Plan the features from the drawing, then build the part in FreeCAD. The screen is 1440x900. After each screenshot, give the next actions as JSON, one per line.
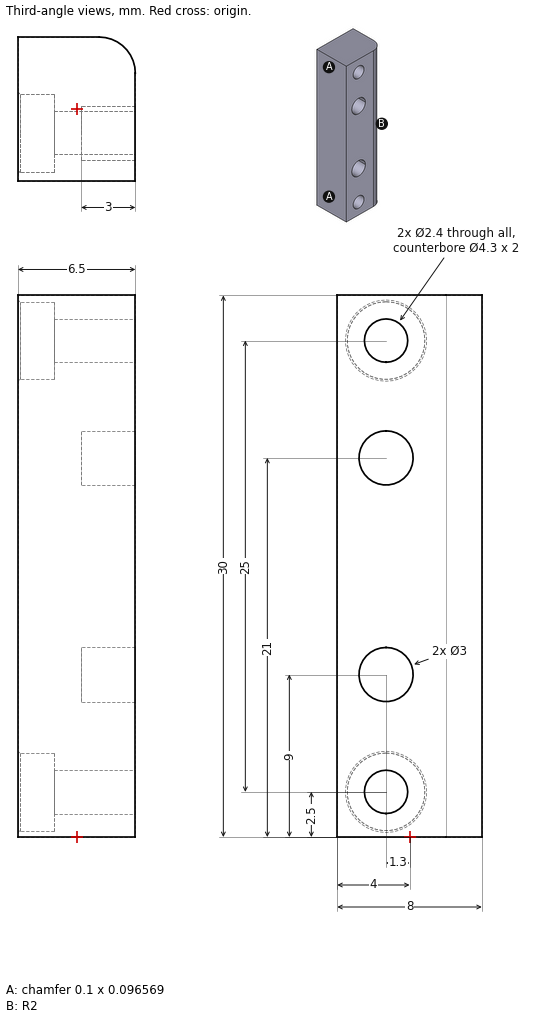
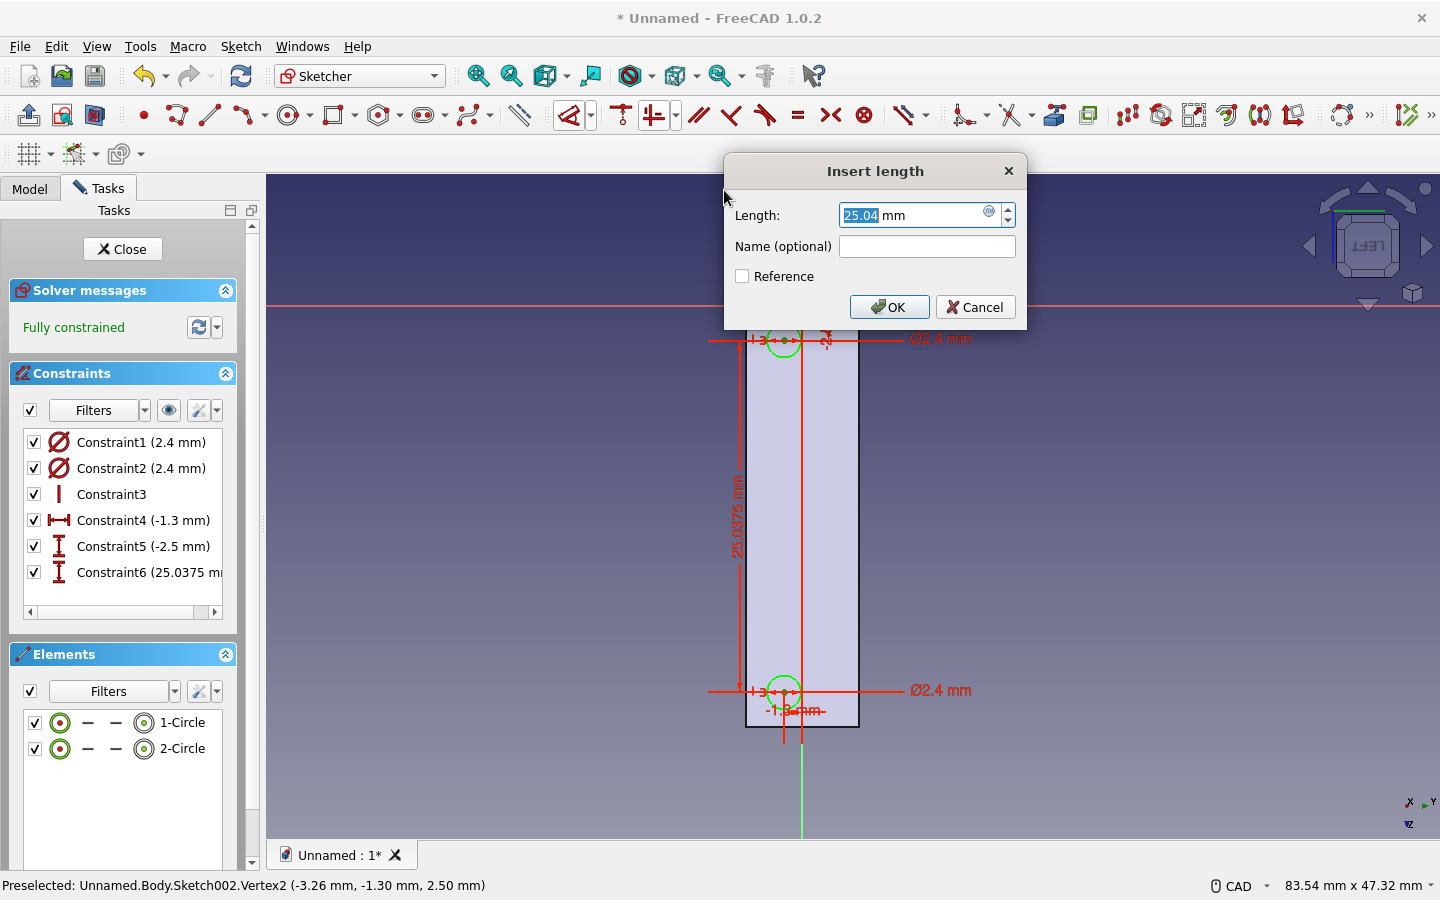
{"action": "type", "text": "25"}
{"action": "key", "text": "Return"}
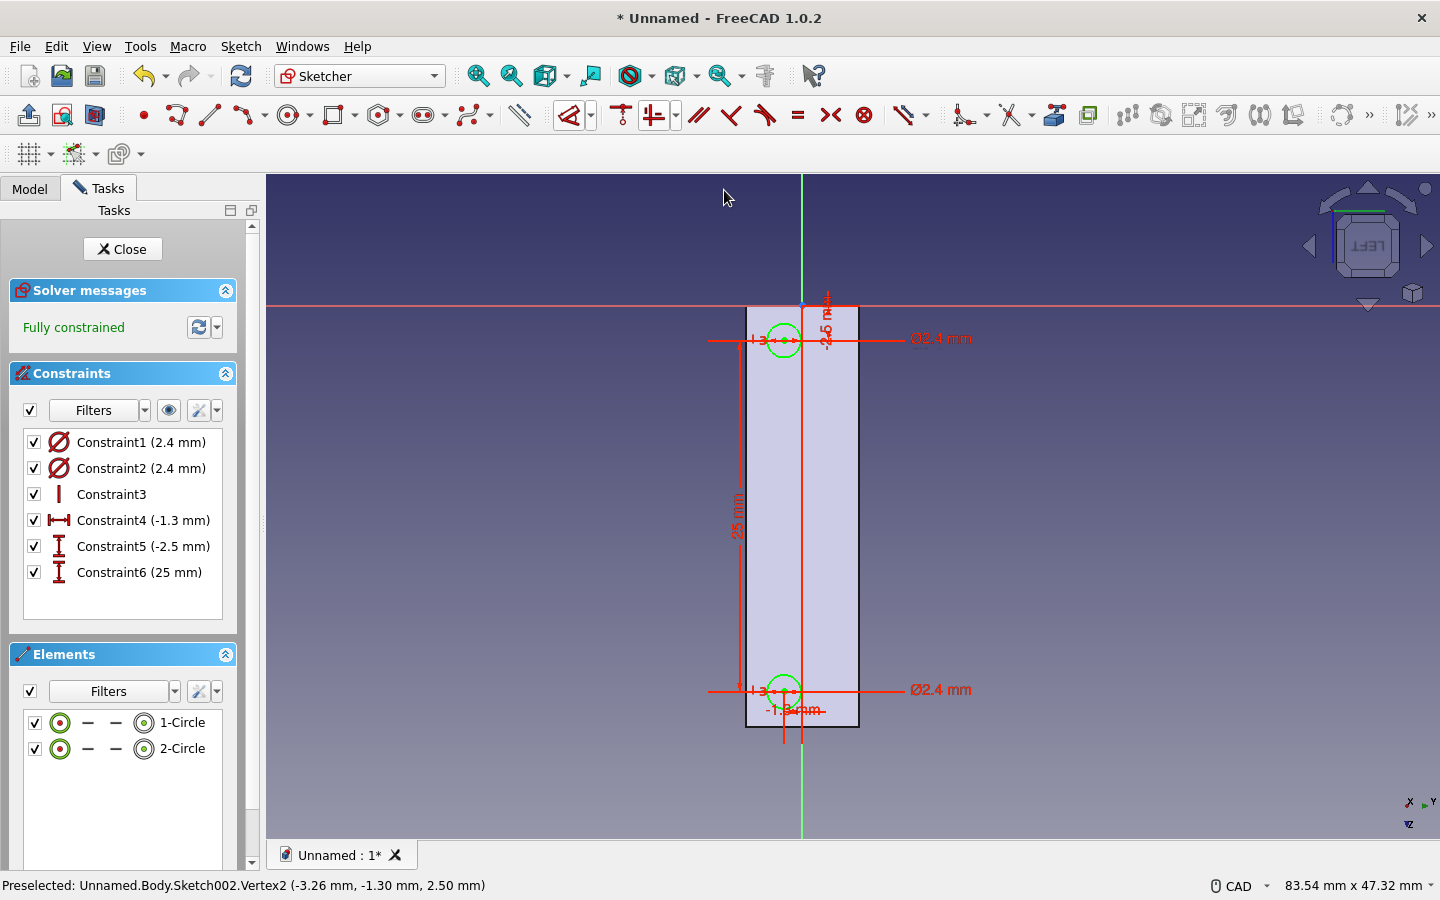
{"action": "left_click", "coordinate": [123, 249]}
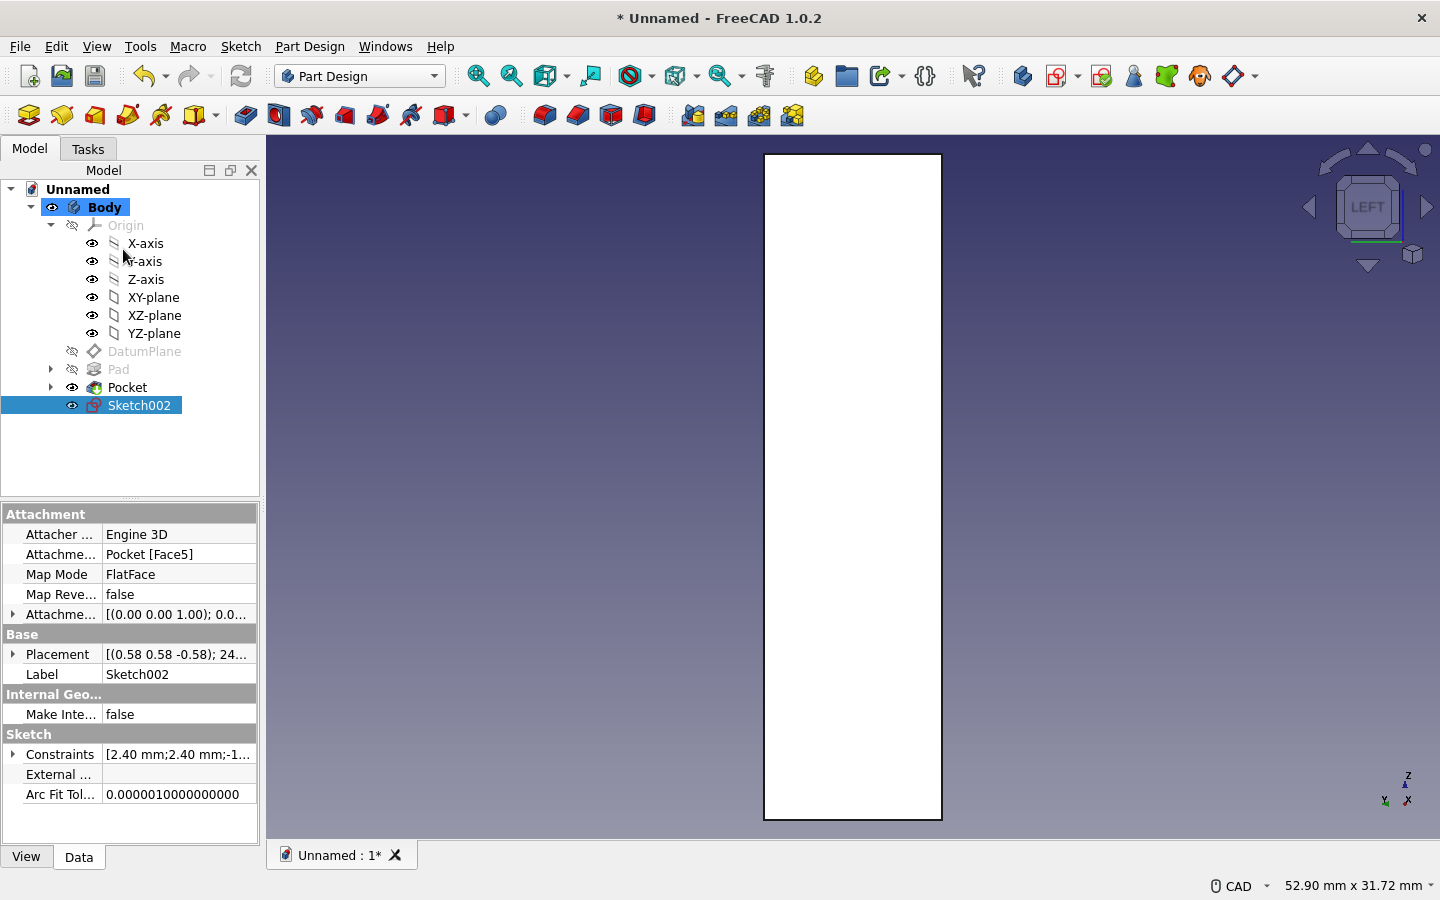
{"action": "left_click", "coordinate": [279, 116]}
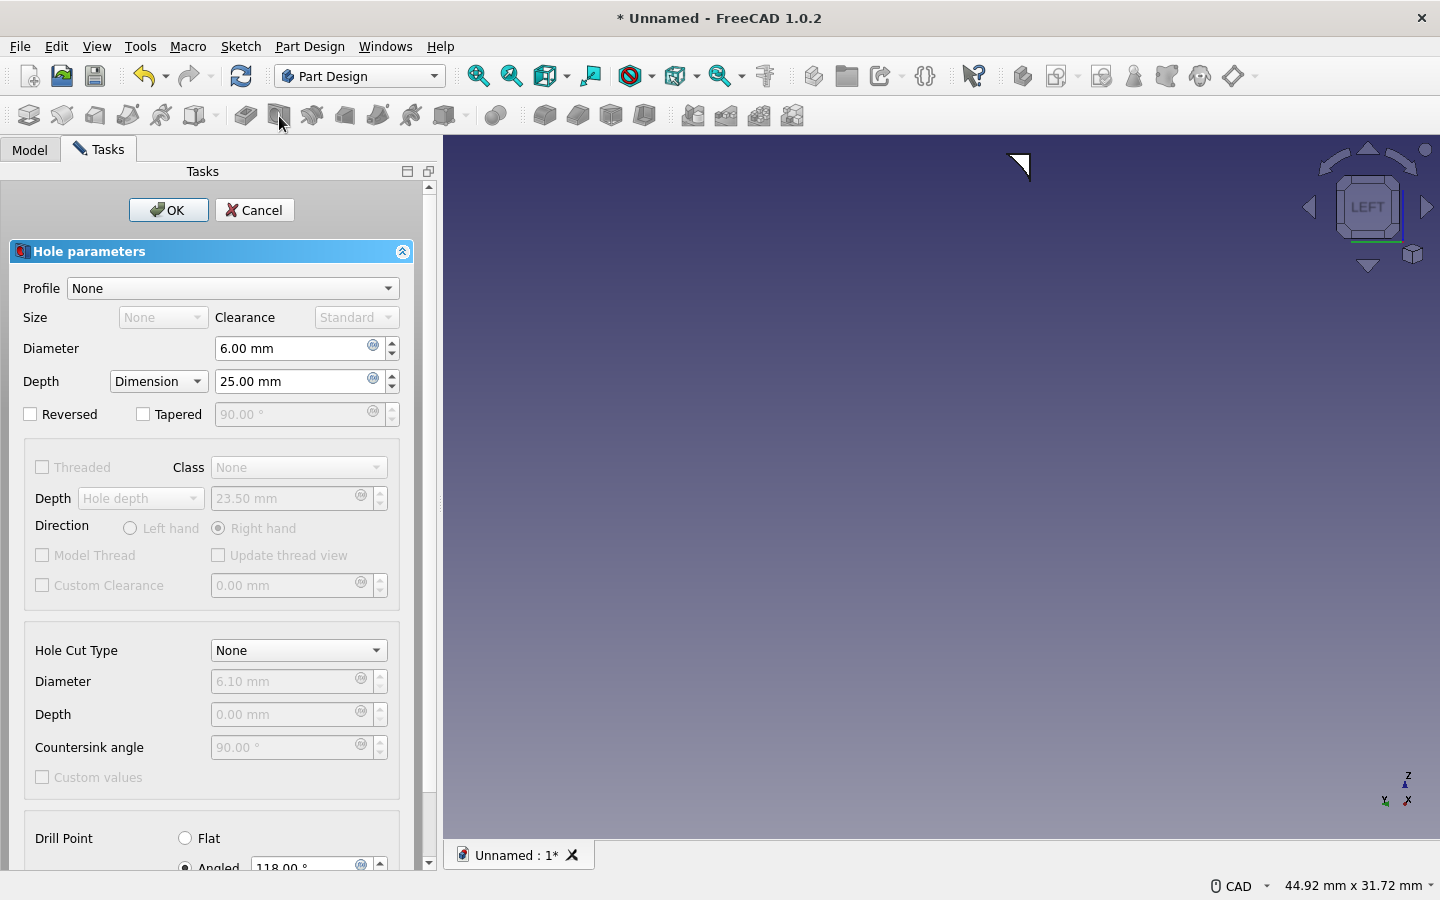
{"action": "triple_click", "coordinate": [300, 348]}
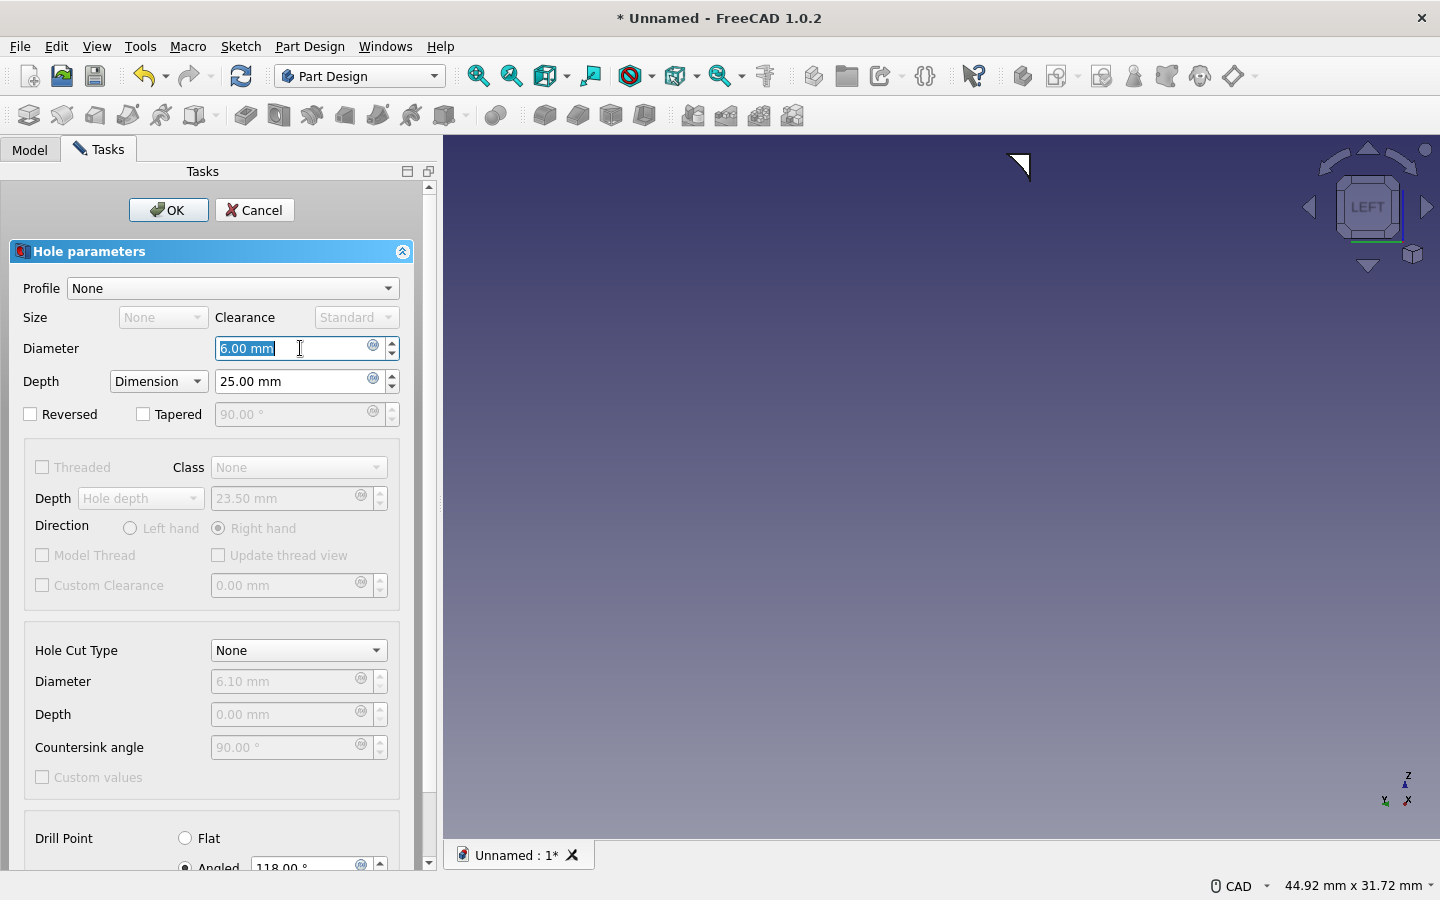
{"action": "type", "text": "2.4"}
{"action": "key", "text": "Tab"}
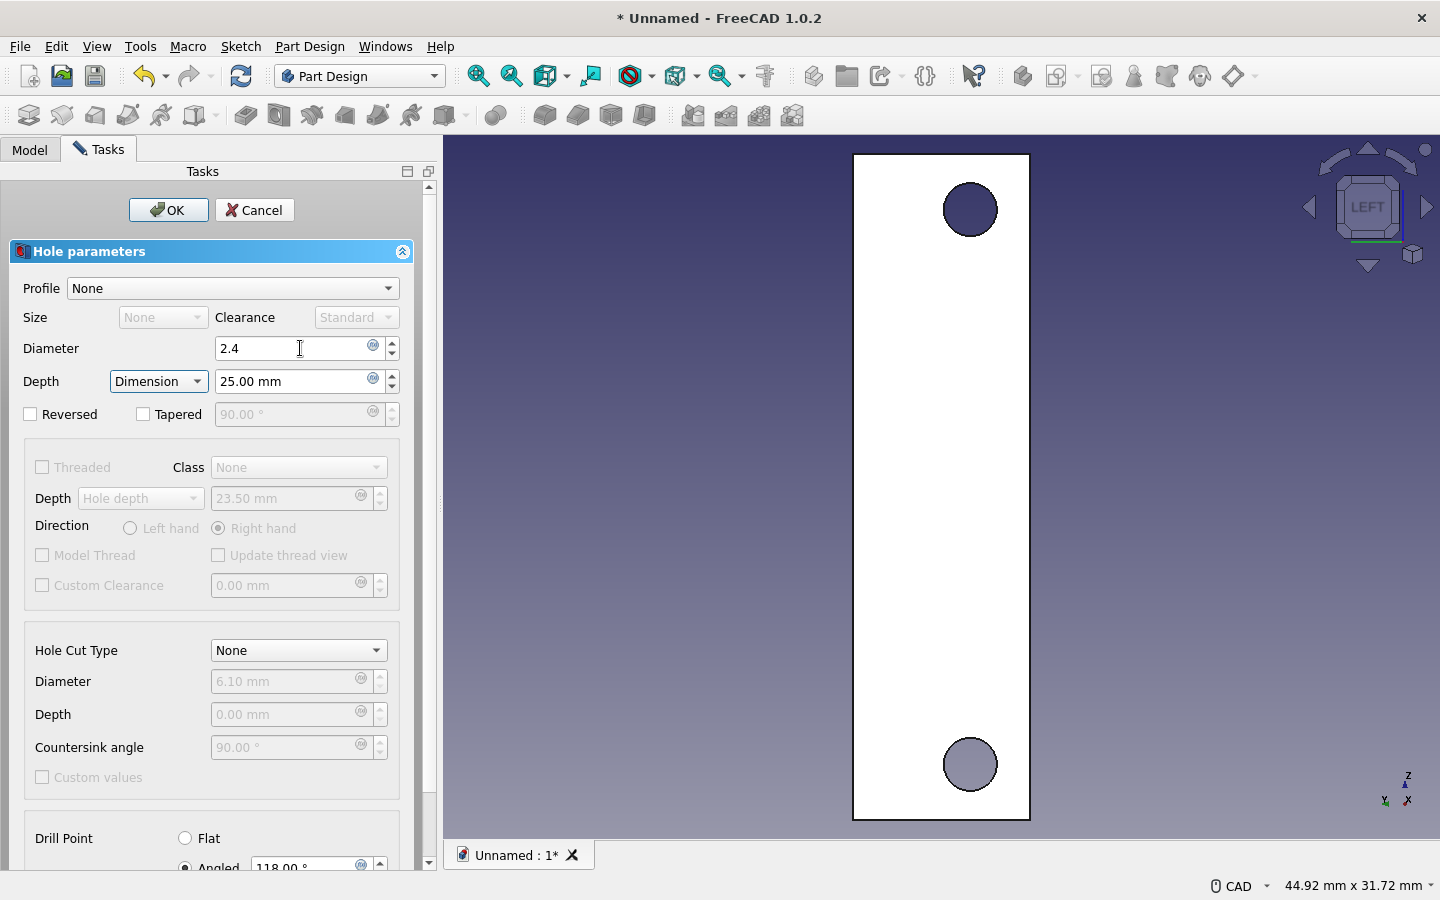
{"action": "left_click", "coordinate": [160, 382]}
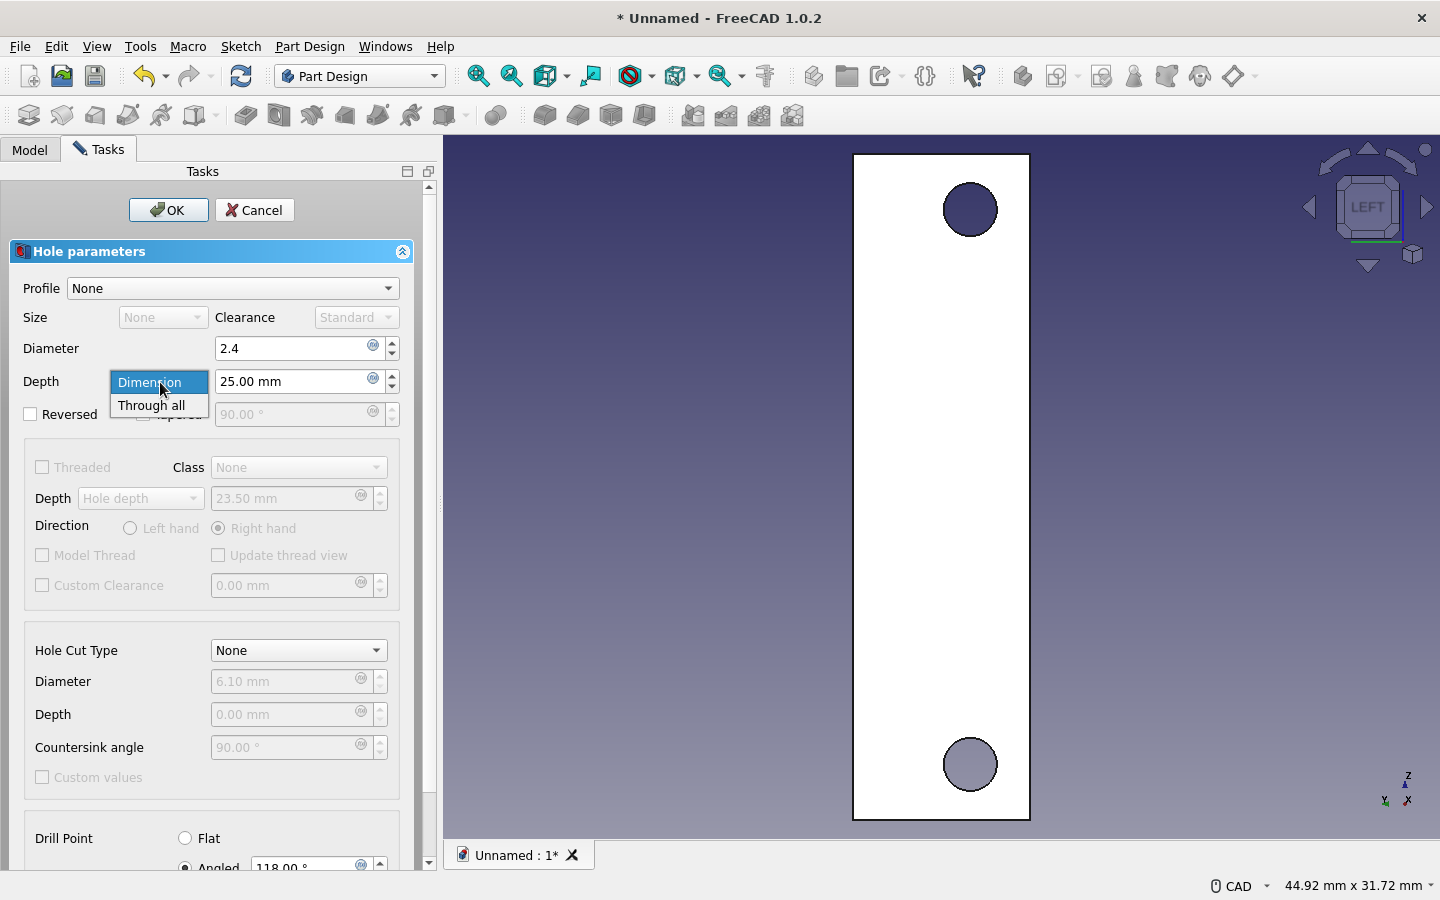
{"action": "left_click", "coordinate": [158, 406]}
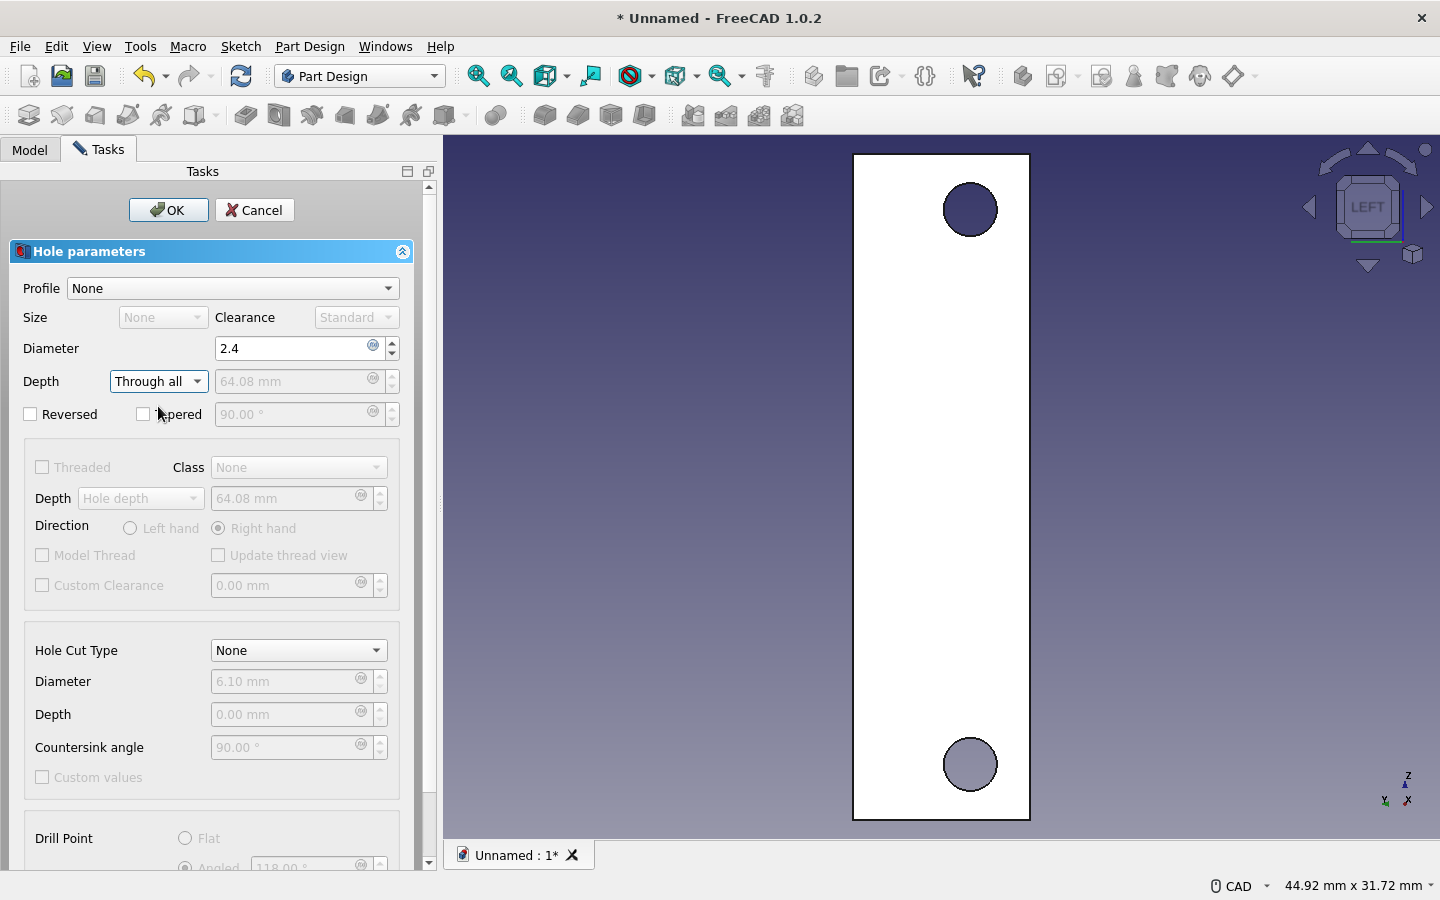
{"action": "left_click", "coordinate": [300, 650]}